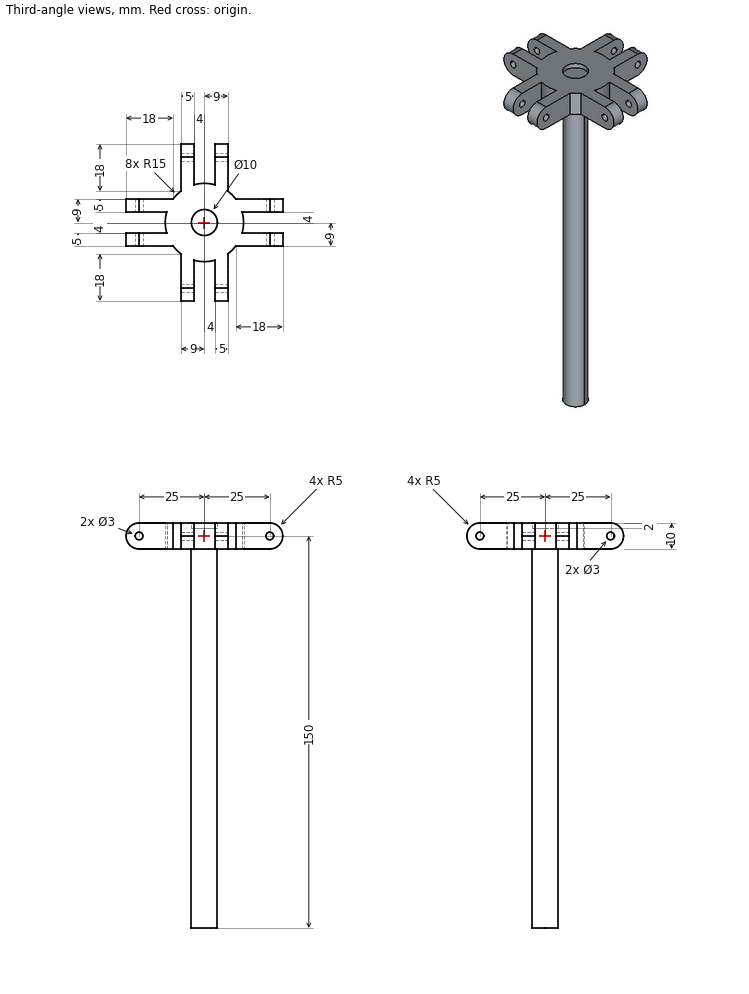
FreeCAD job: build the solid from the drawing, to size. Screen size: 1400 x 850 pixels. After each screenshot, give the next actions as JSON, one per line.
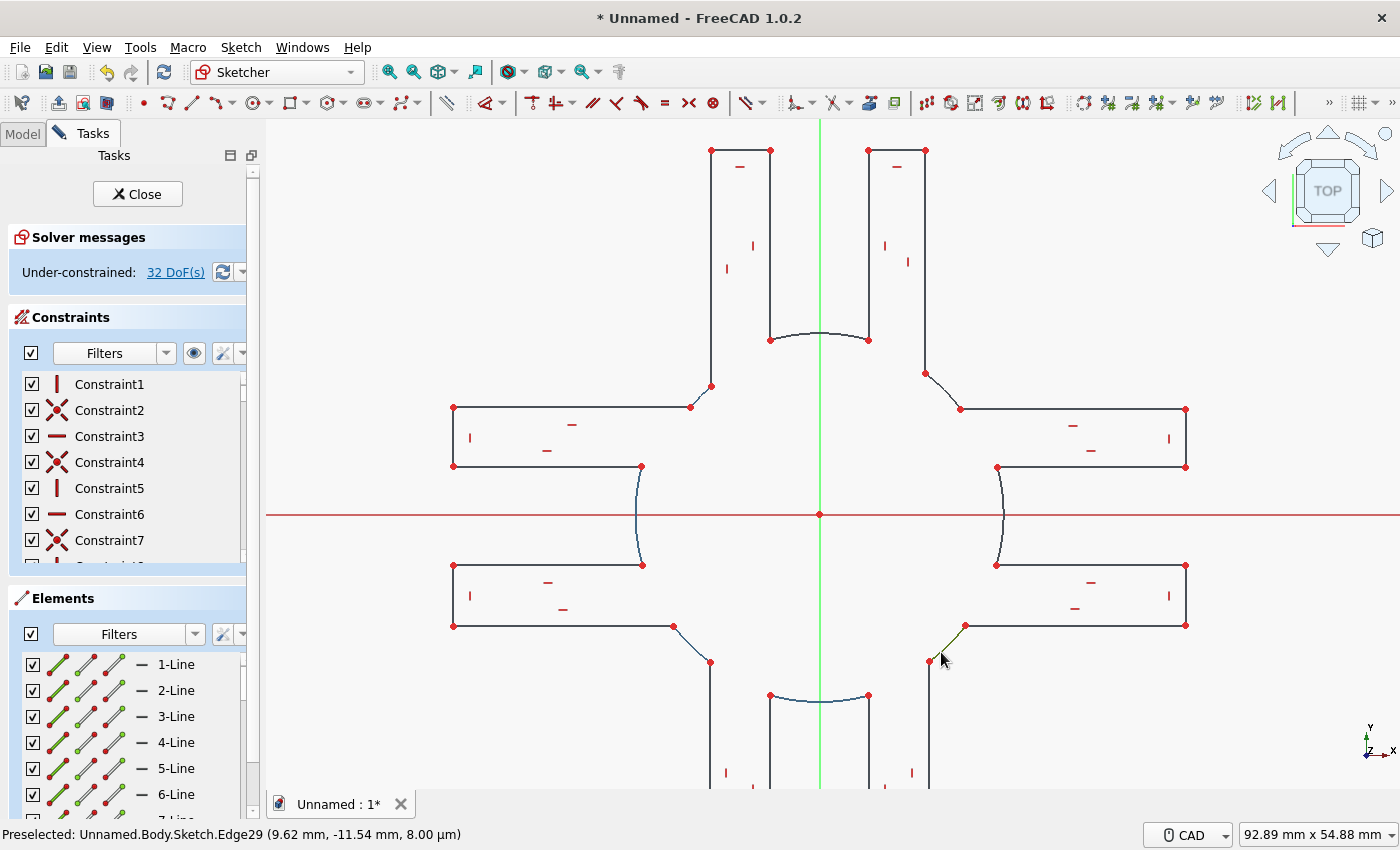
{"action": "left_click", "coordinate": [1002, 536]}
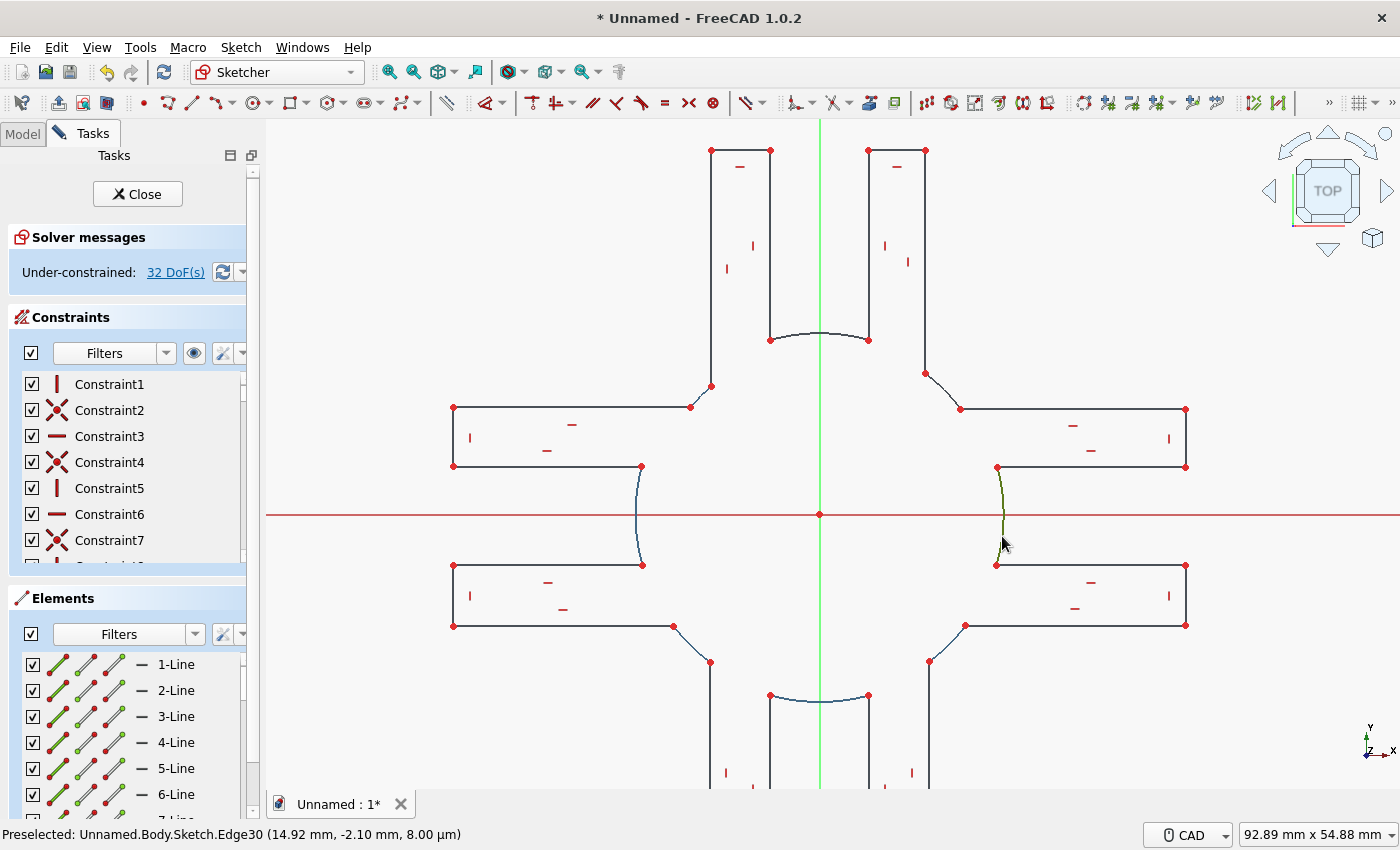
{"action": "left_click", "coordinate": [951, 397]}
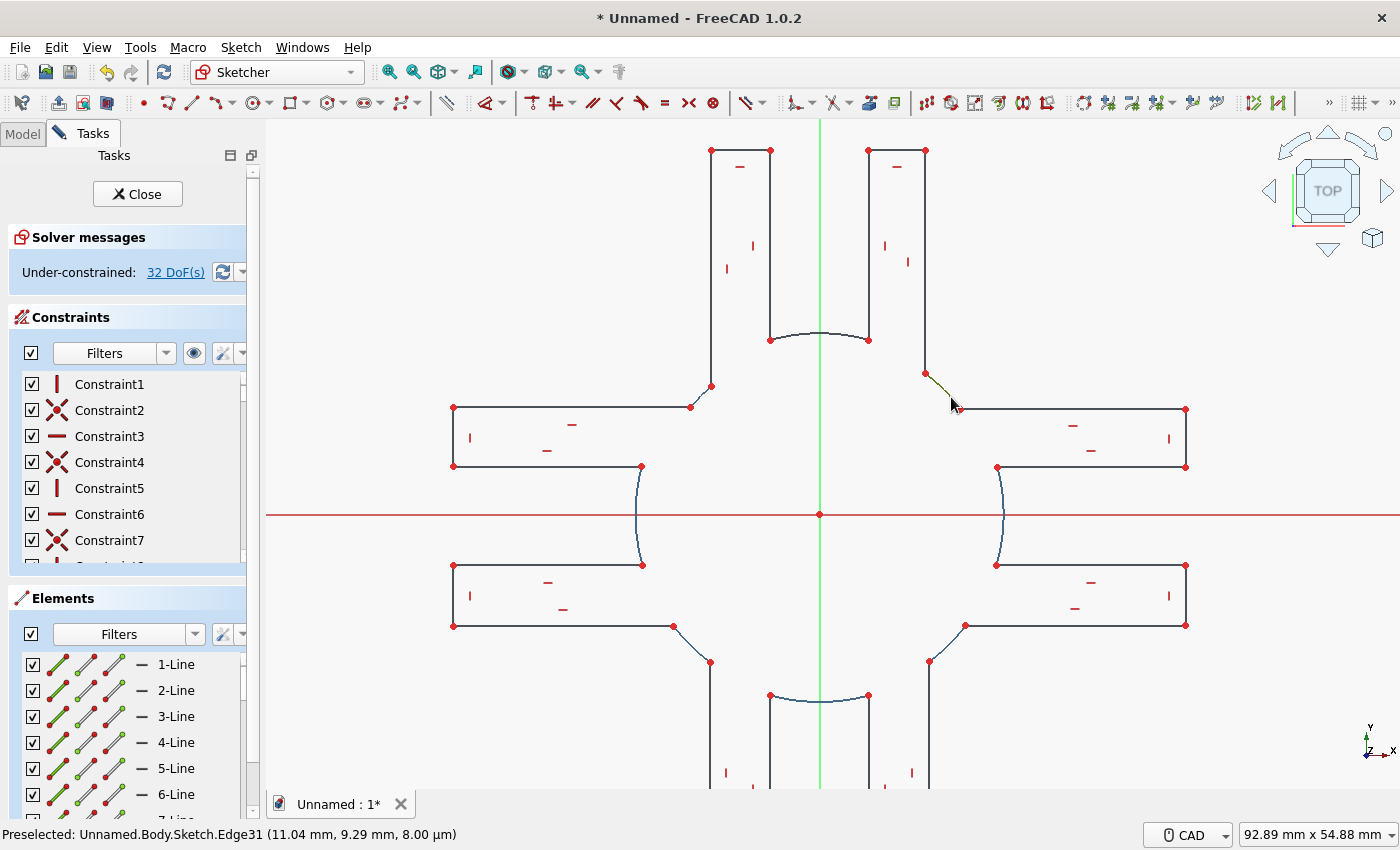
{"action": "left_click", "coordinate": [839, 334]}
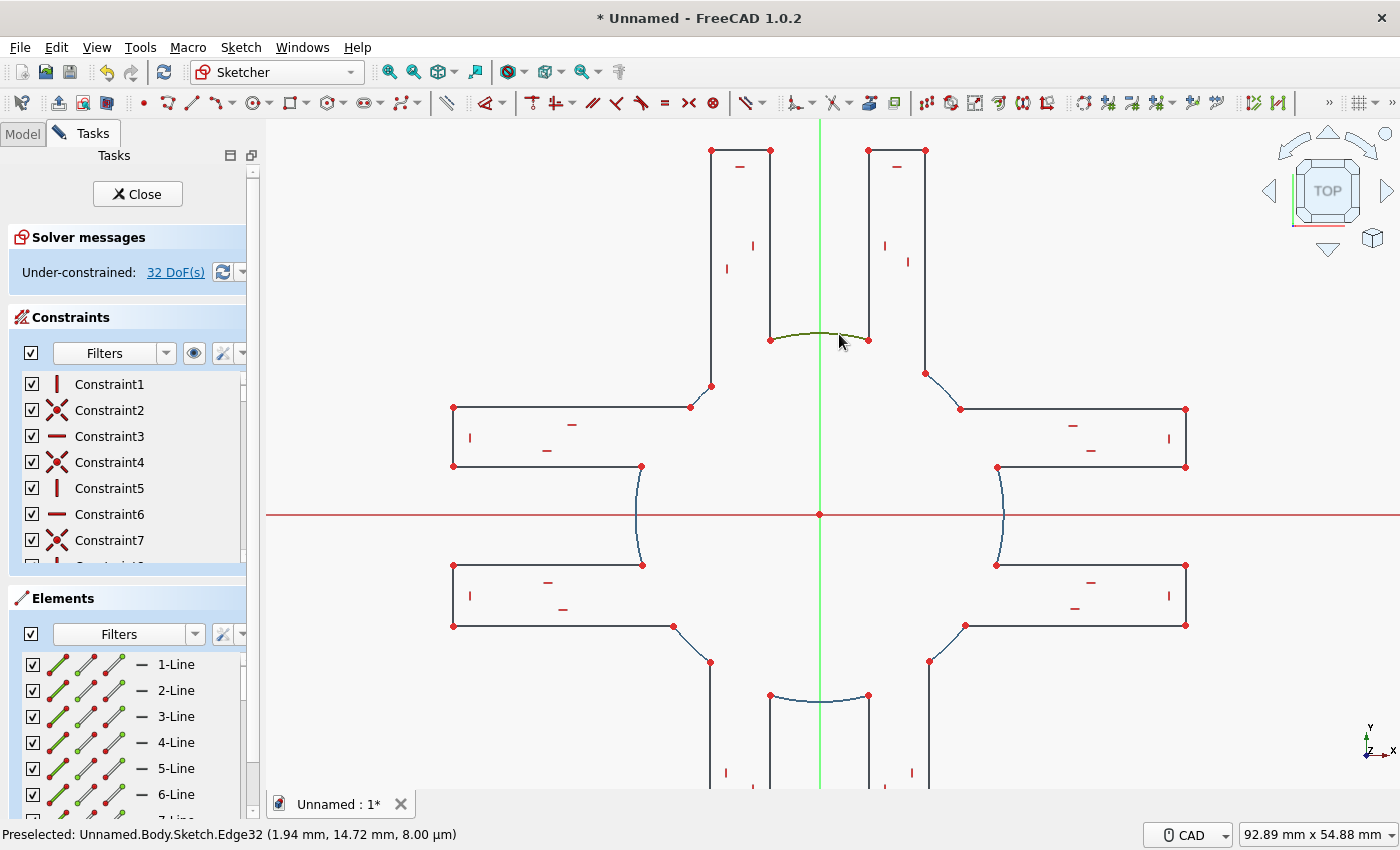
{"action": "key", "text": "e"}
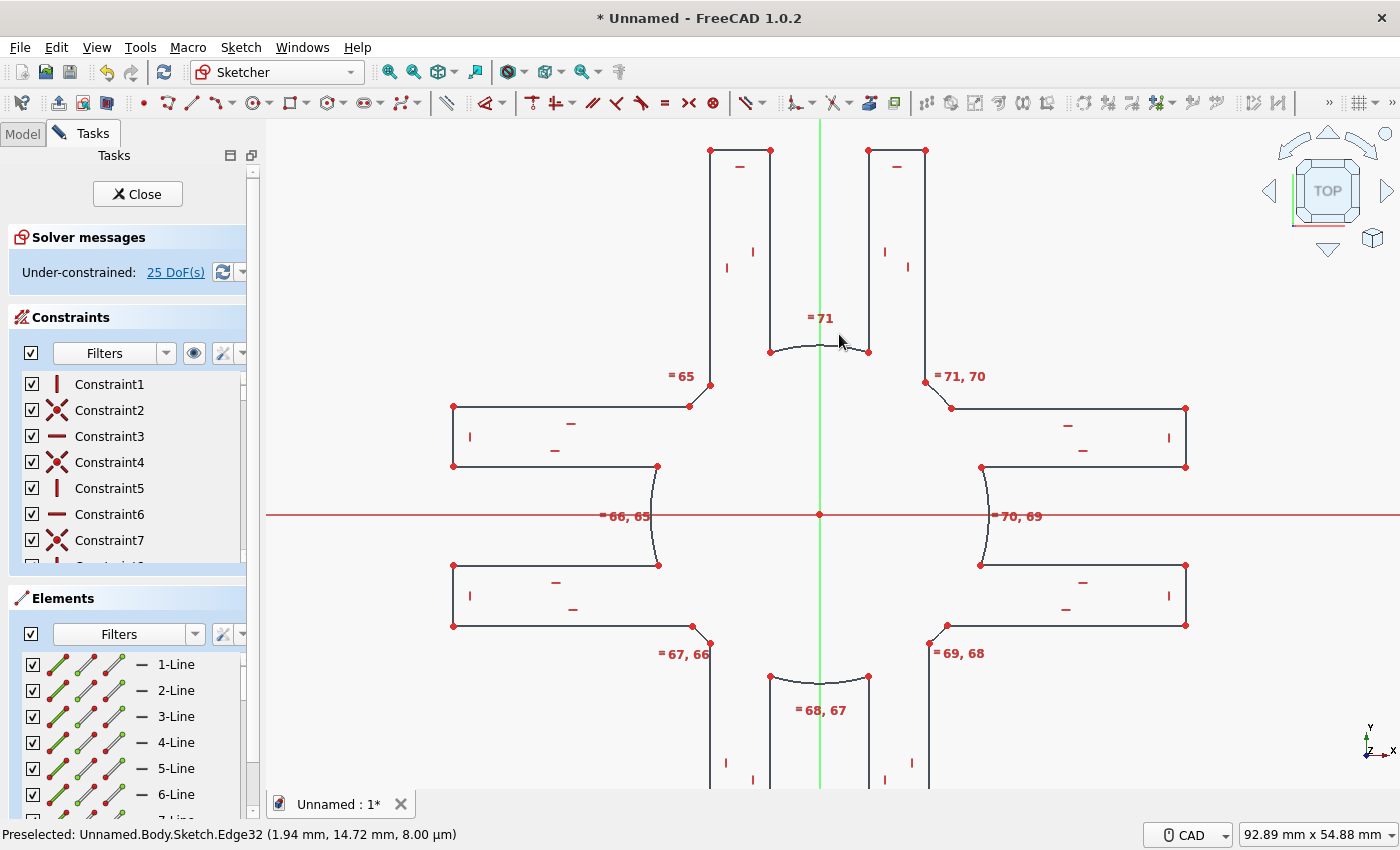
{"action": "key", "text": "d"}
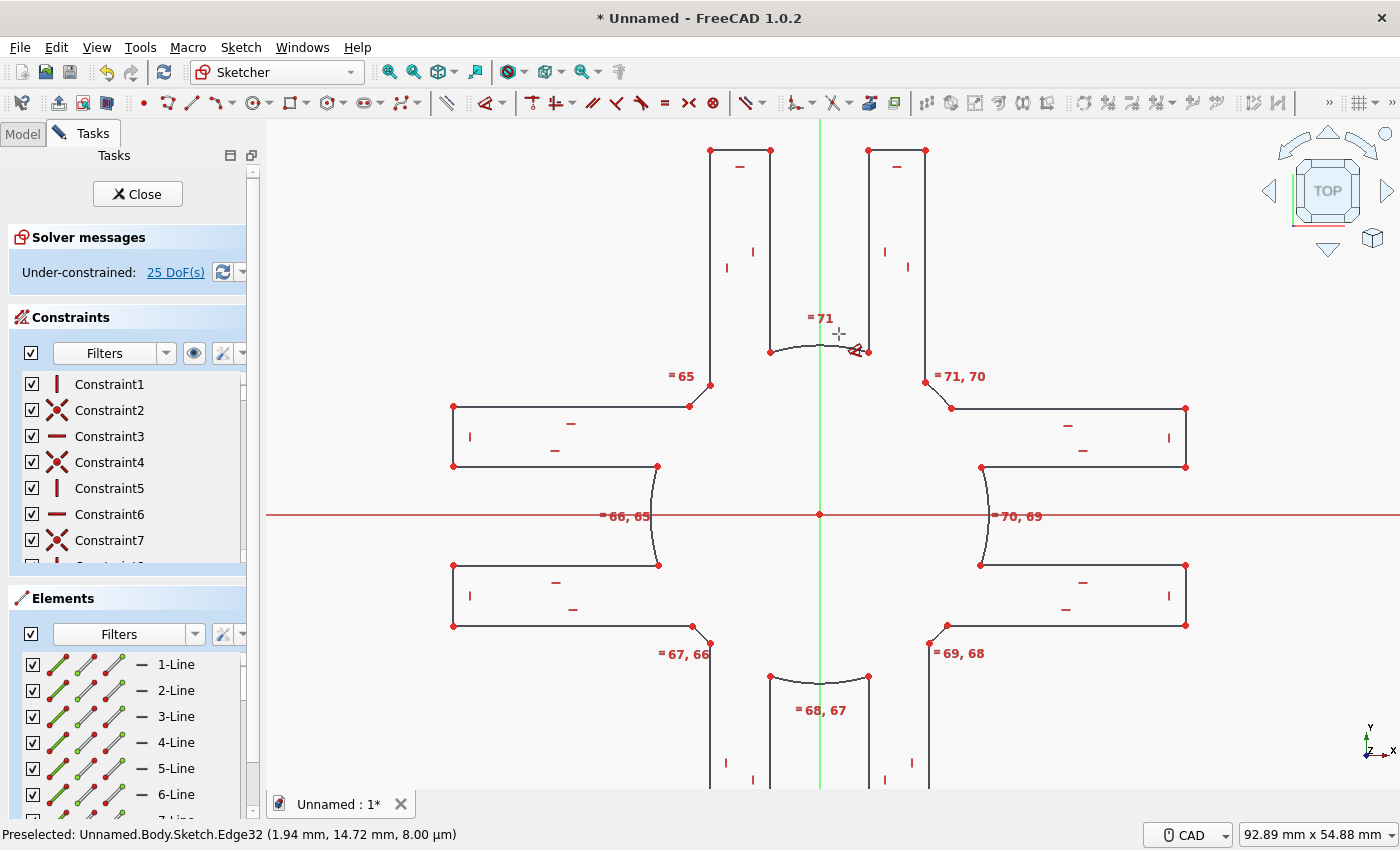
{"action": "left_click", "coordinate": [699, 396]}
{"action": "left_click", "coordinate": [676, 374]}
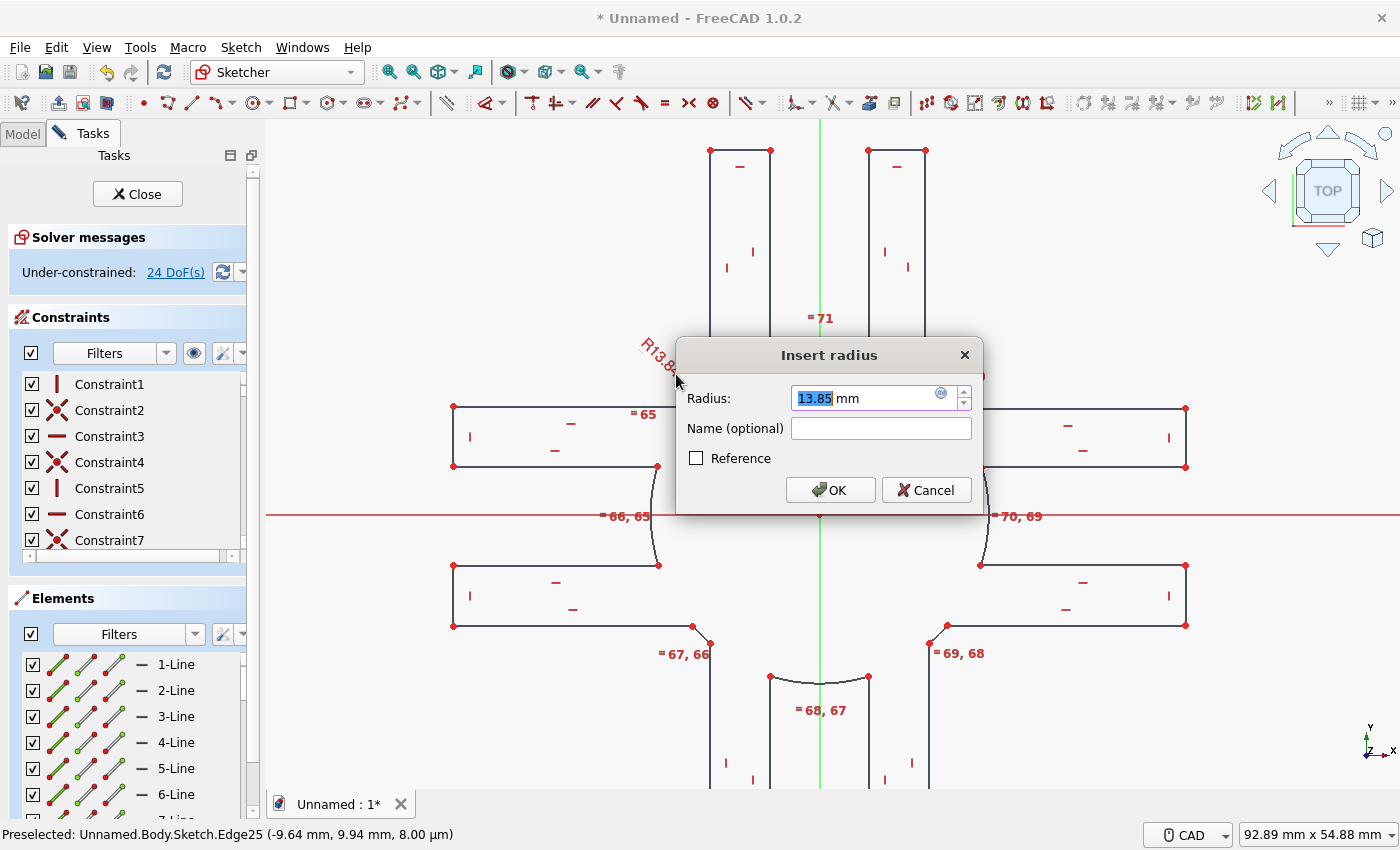
{"action": "type", "text": "15"}
{"action": "key", "text": "Return"}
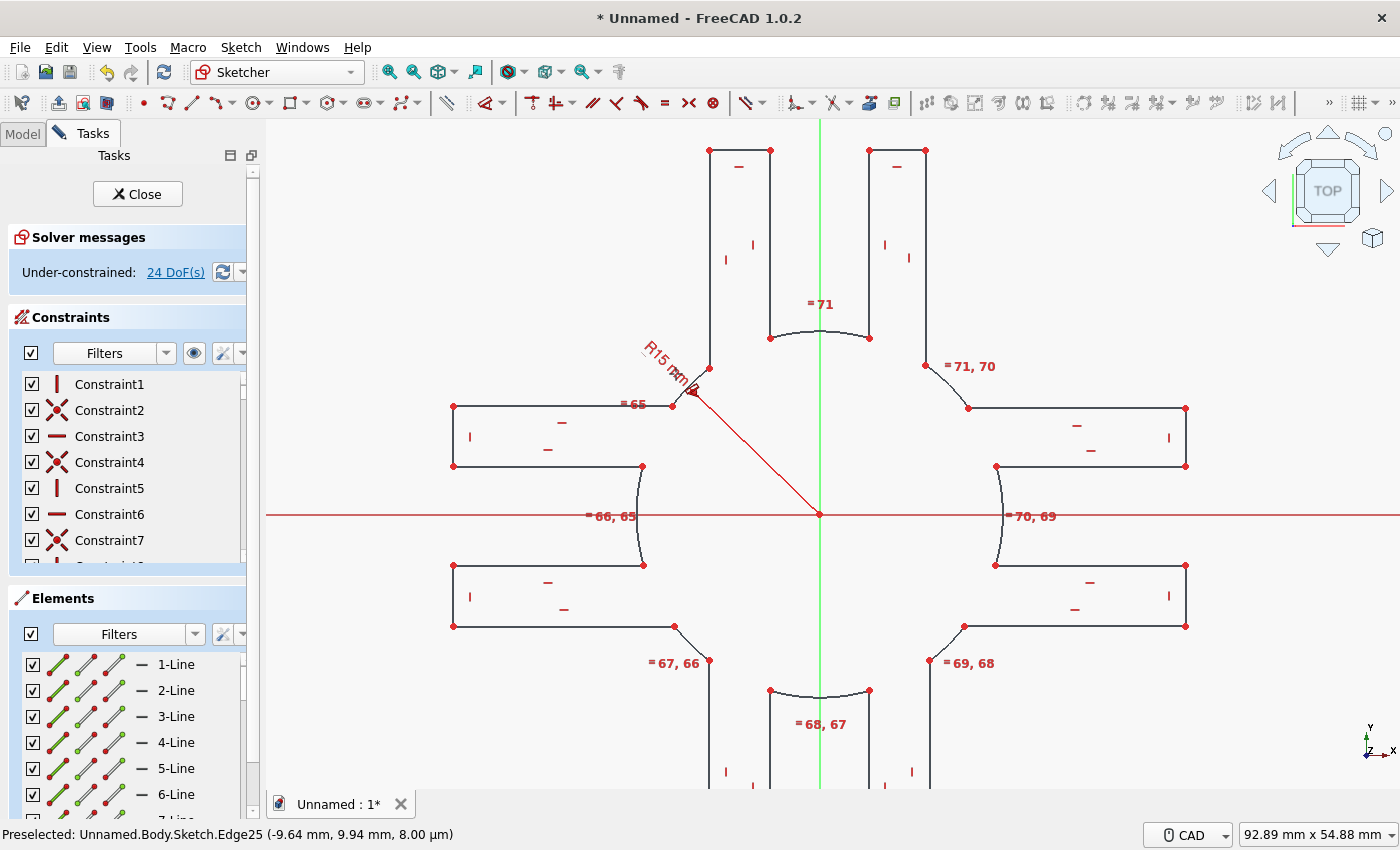
{"action": "left_click", "coordinate": [752, 150]}
{"action": "left_click", "coordinate": [740, 184]}